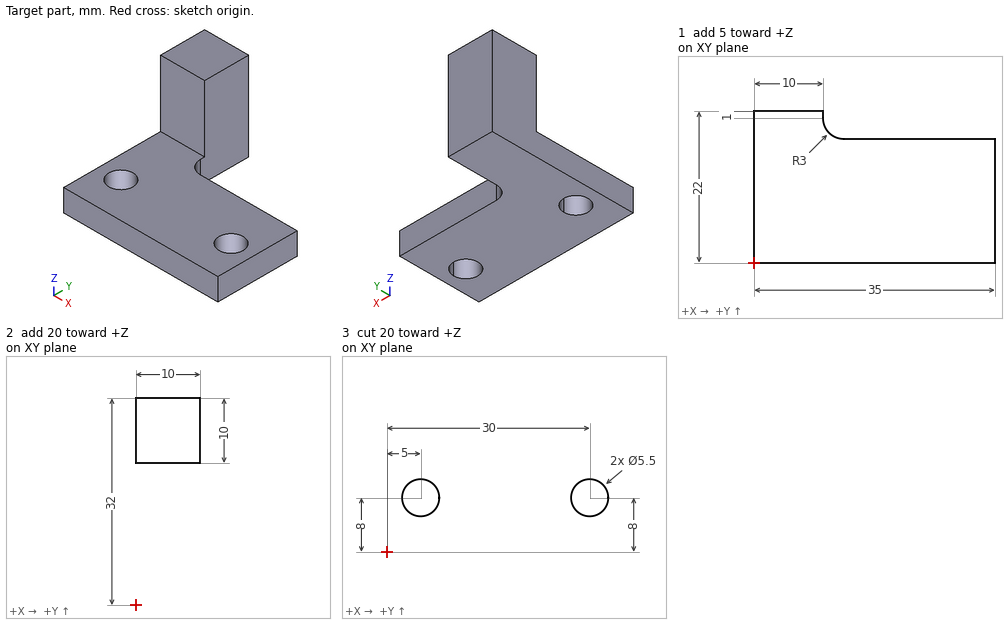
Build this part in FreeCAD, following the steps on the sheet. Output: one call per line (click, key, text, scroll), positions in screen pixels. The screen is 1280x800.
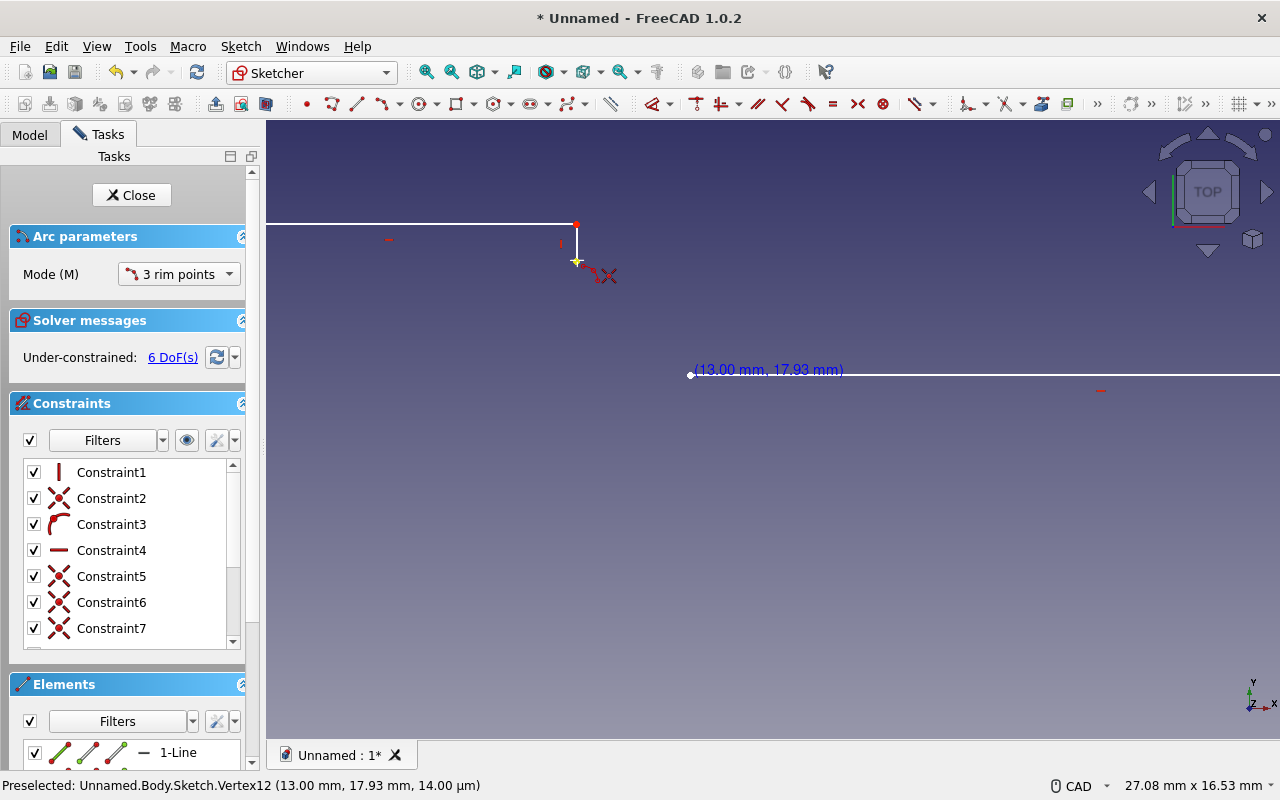
click(577, 262)
click(611, 340)
key(Escape)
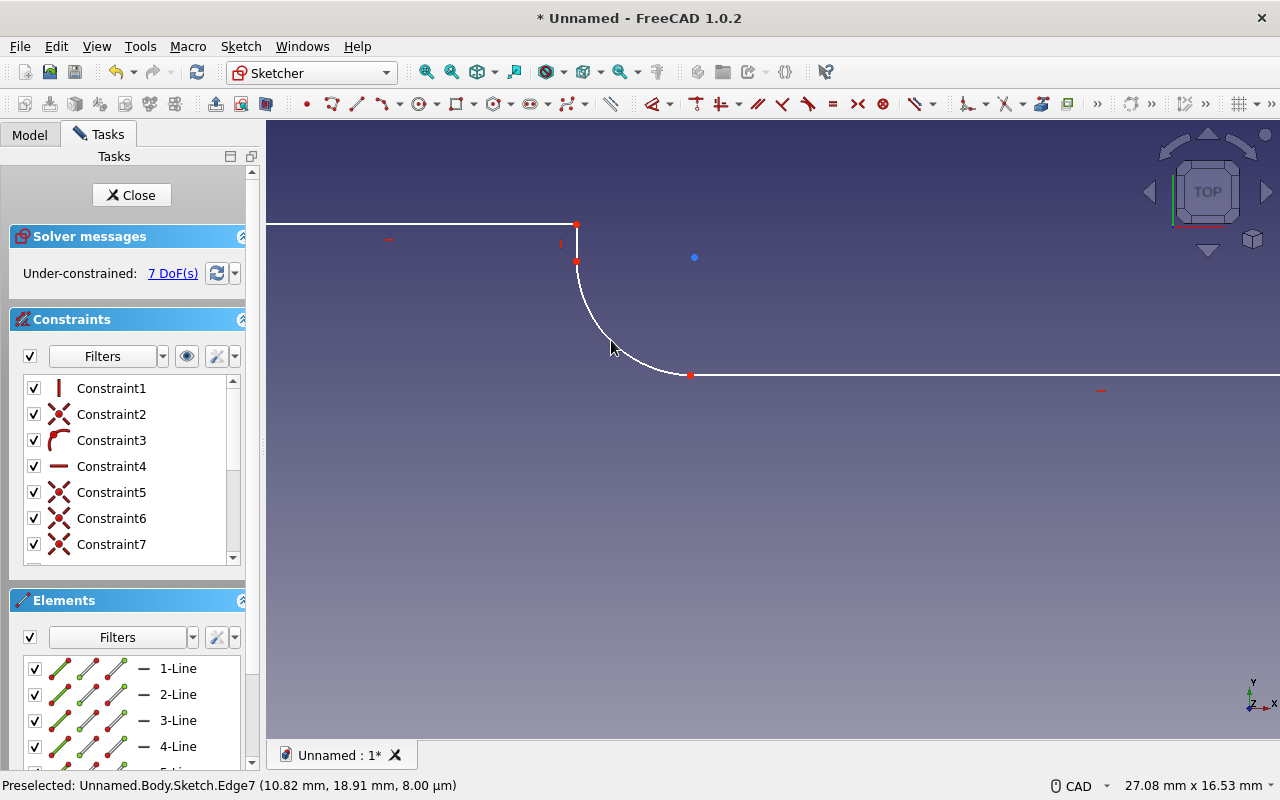
click(577, 251)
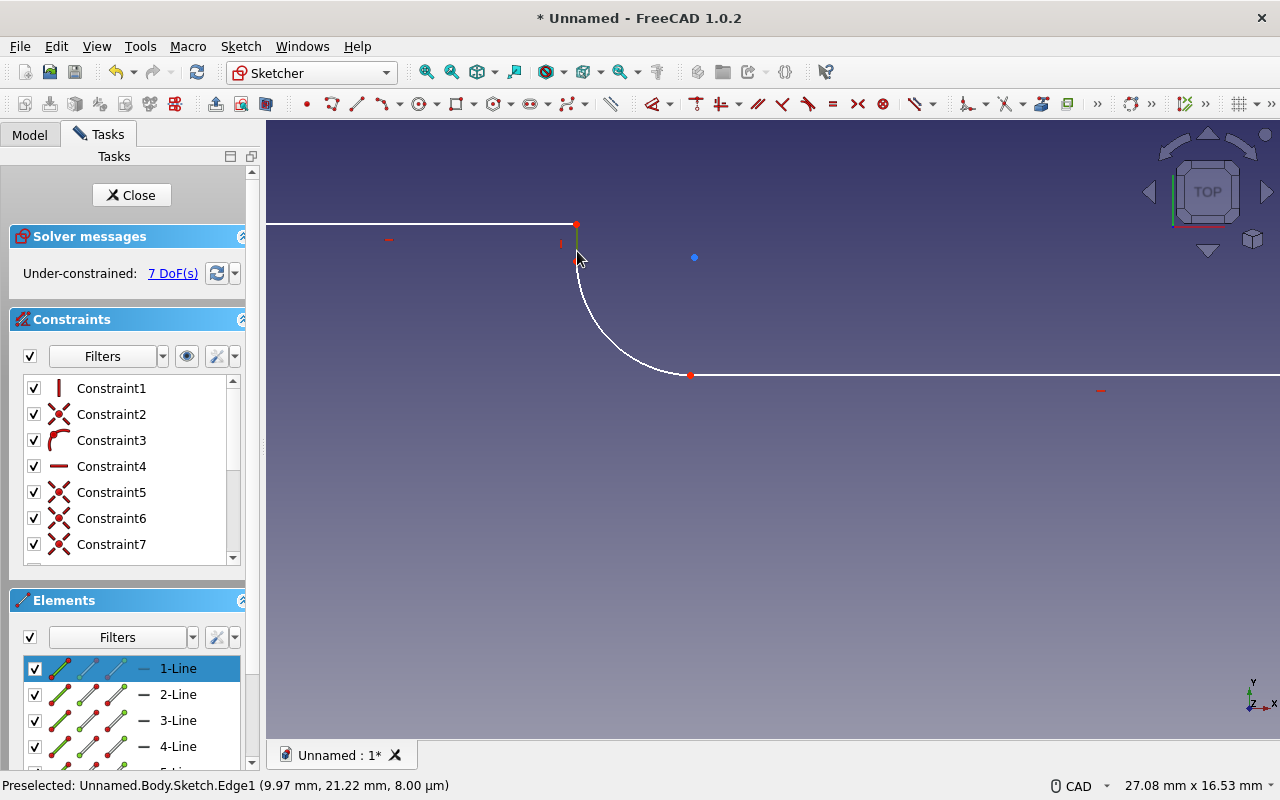
click(590, 313)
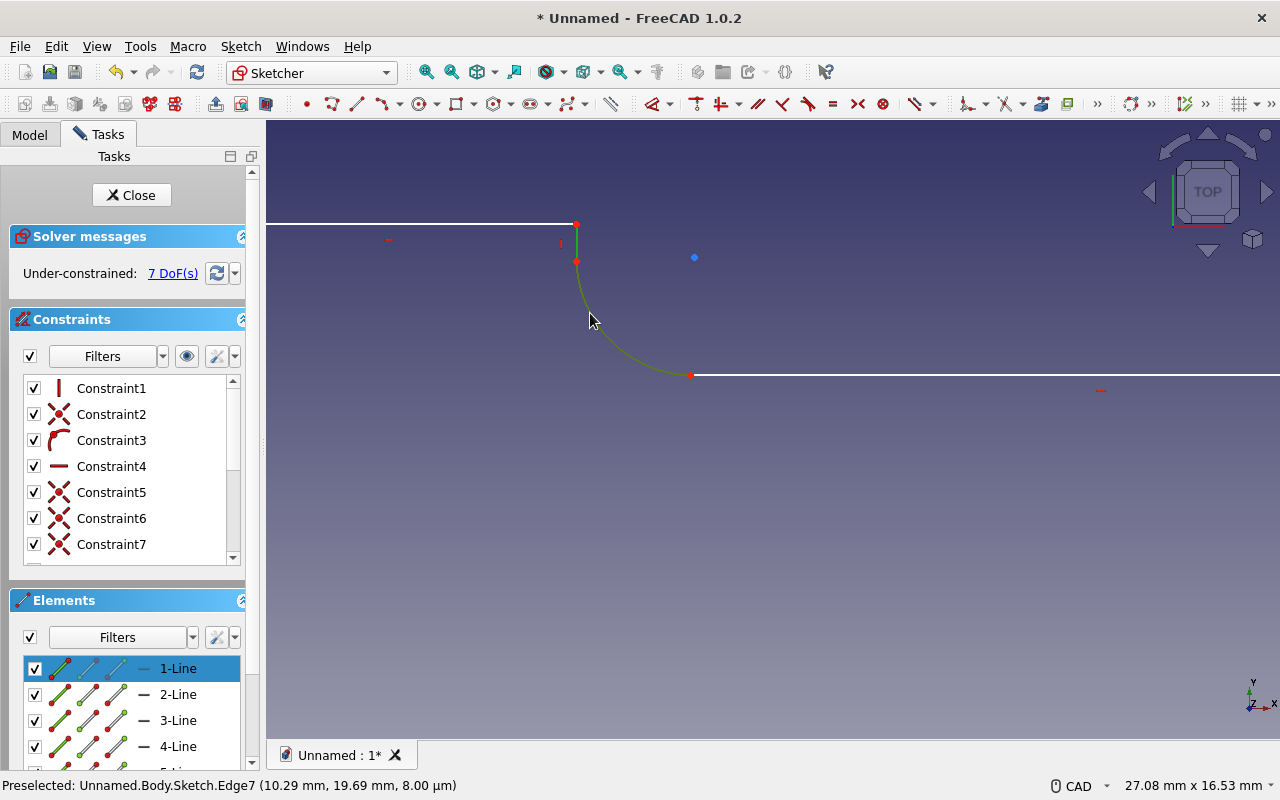
click(808, 104)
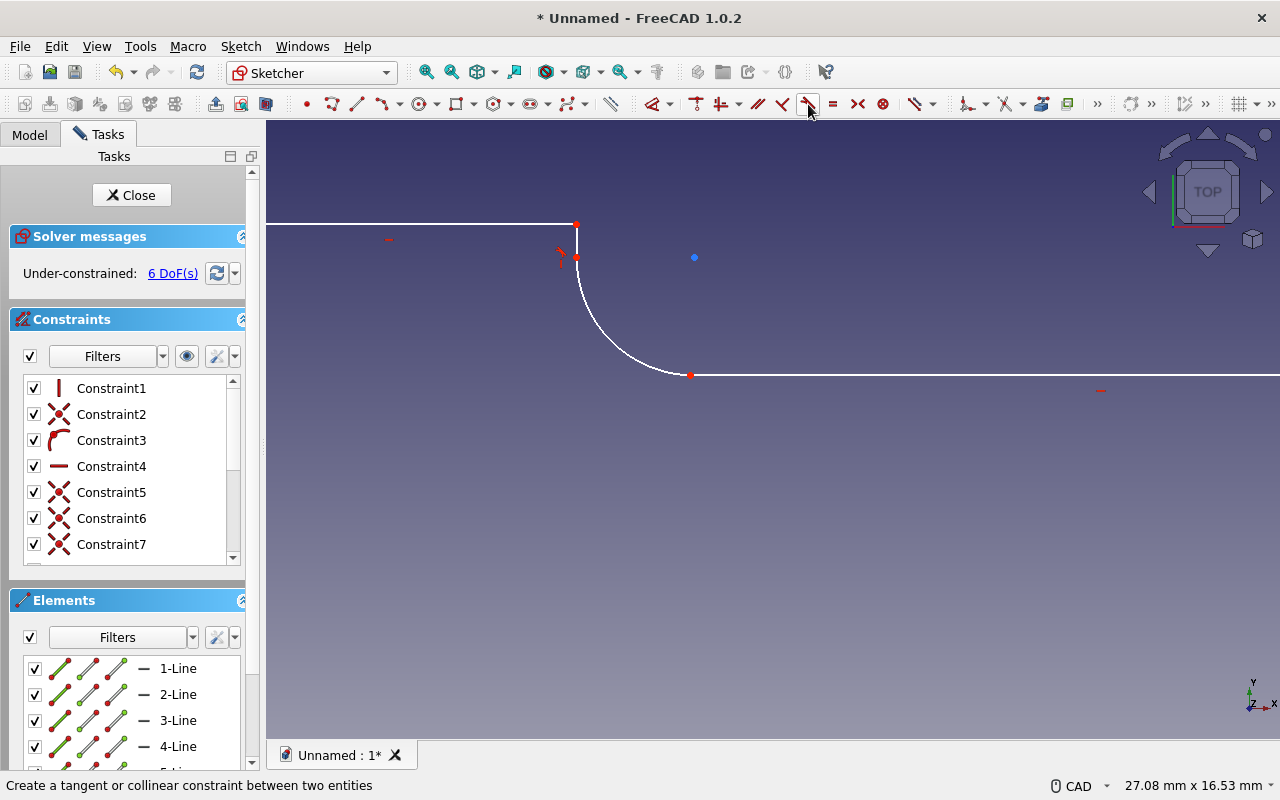
click(937, 375)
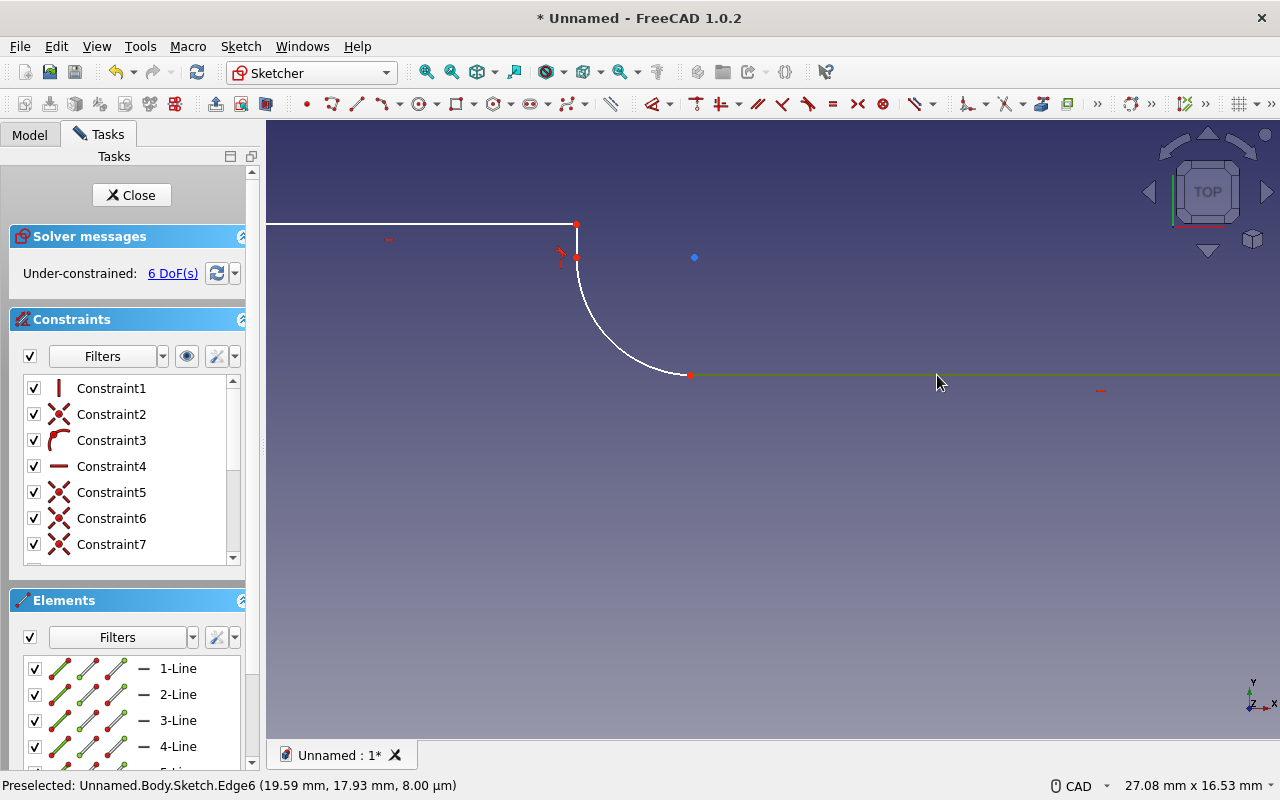
click(589, 310)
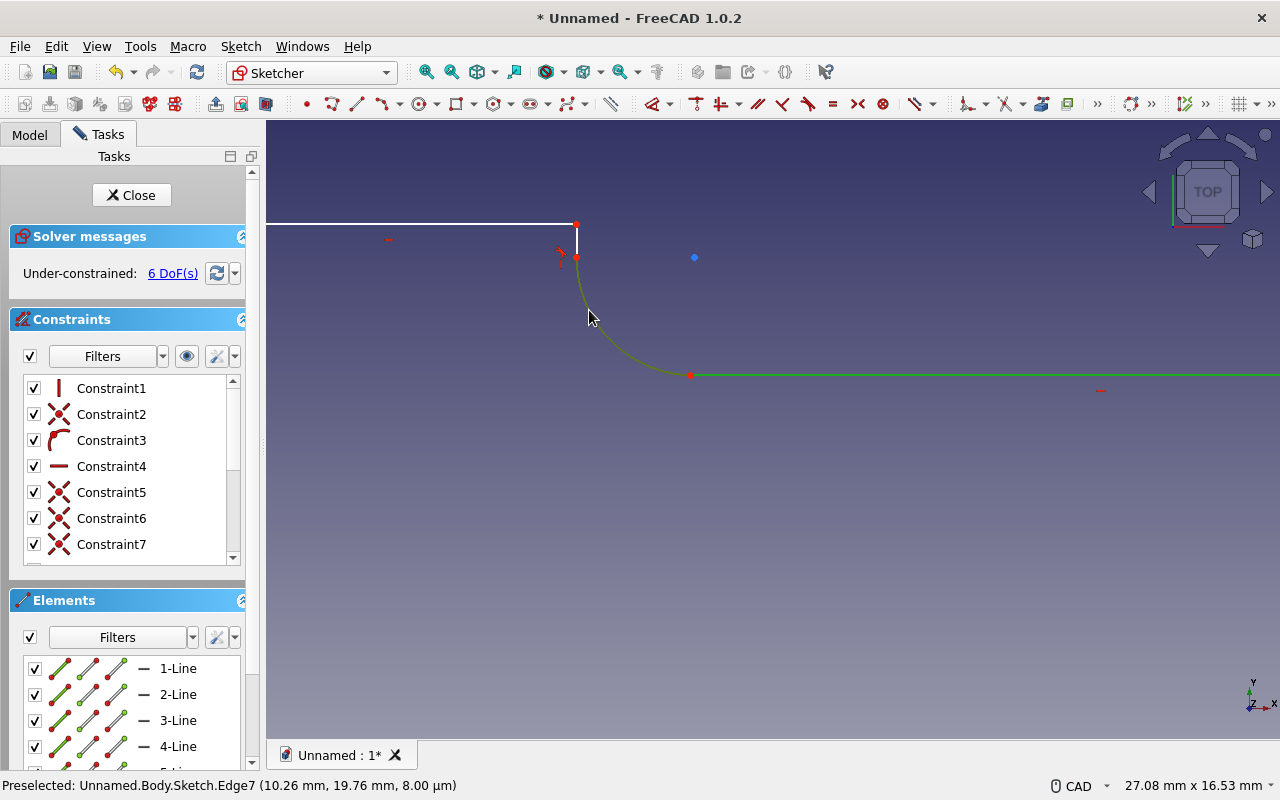
click(808, 104)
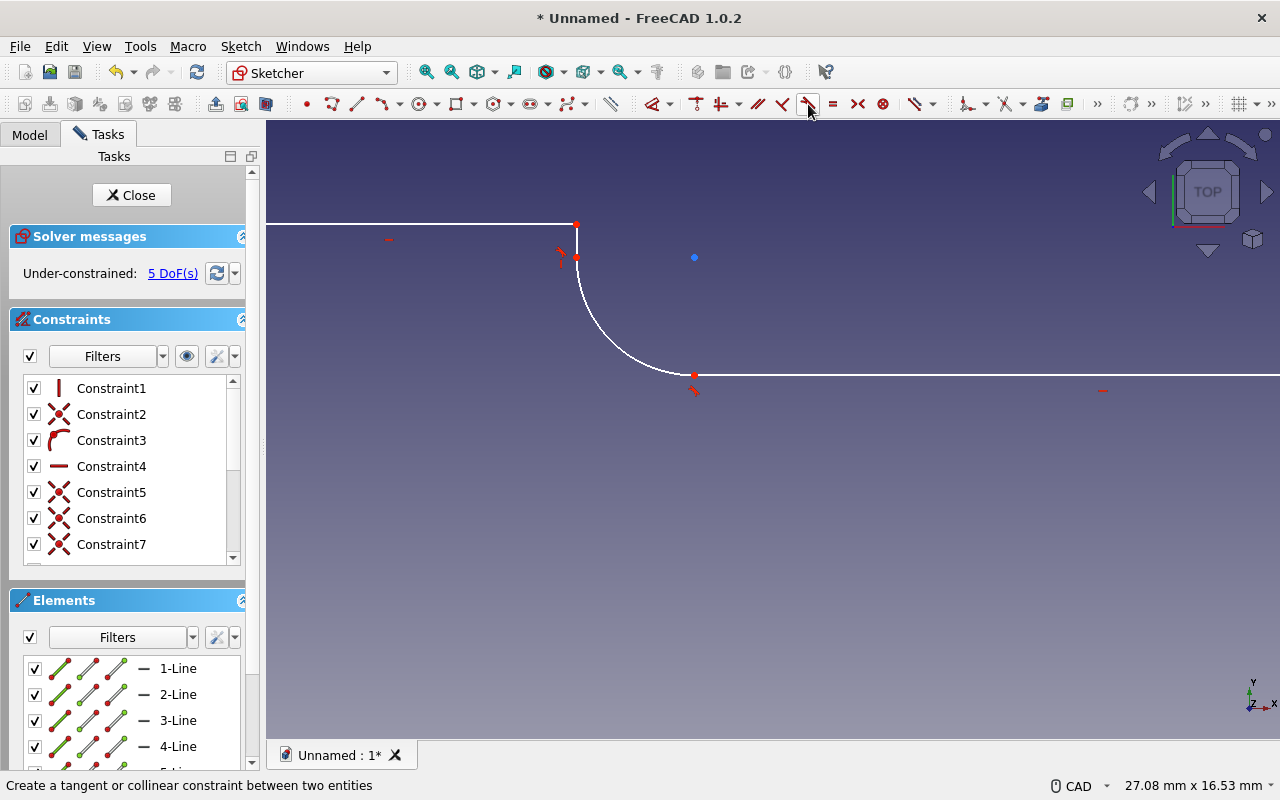
click(652, 104)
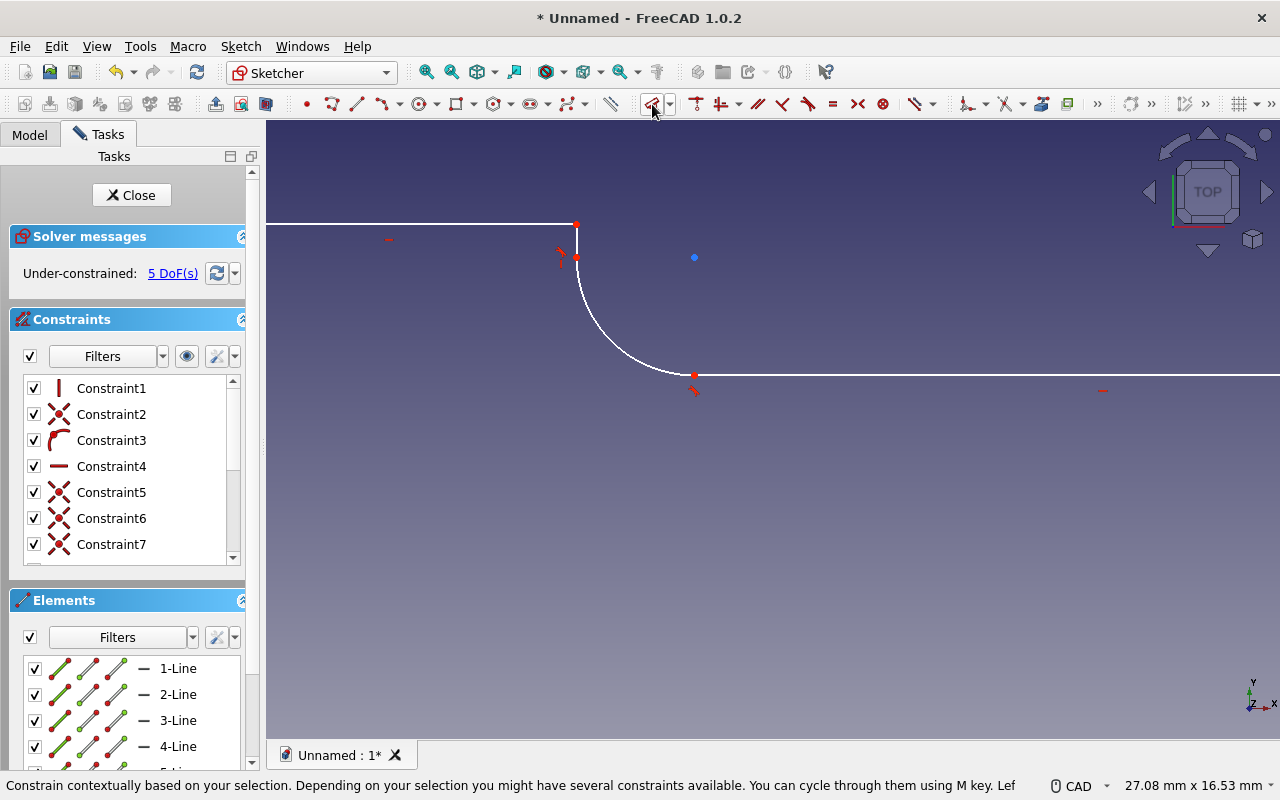
click(590, 311)
click(561, 326)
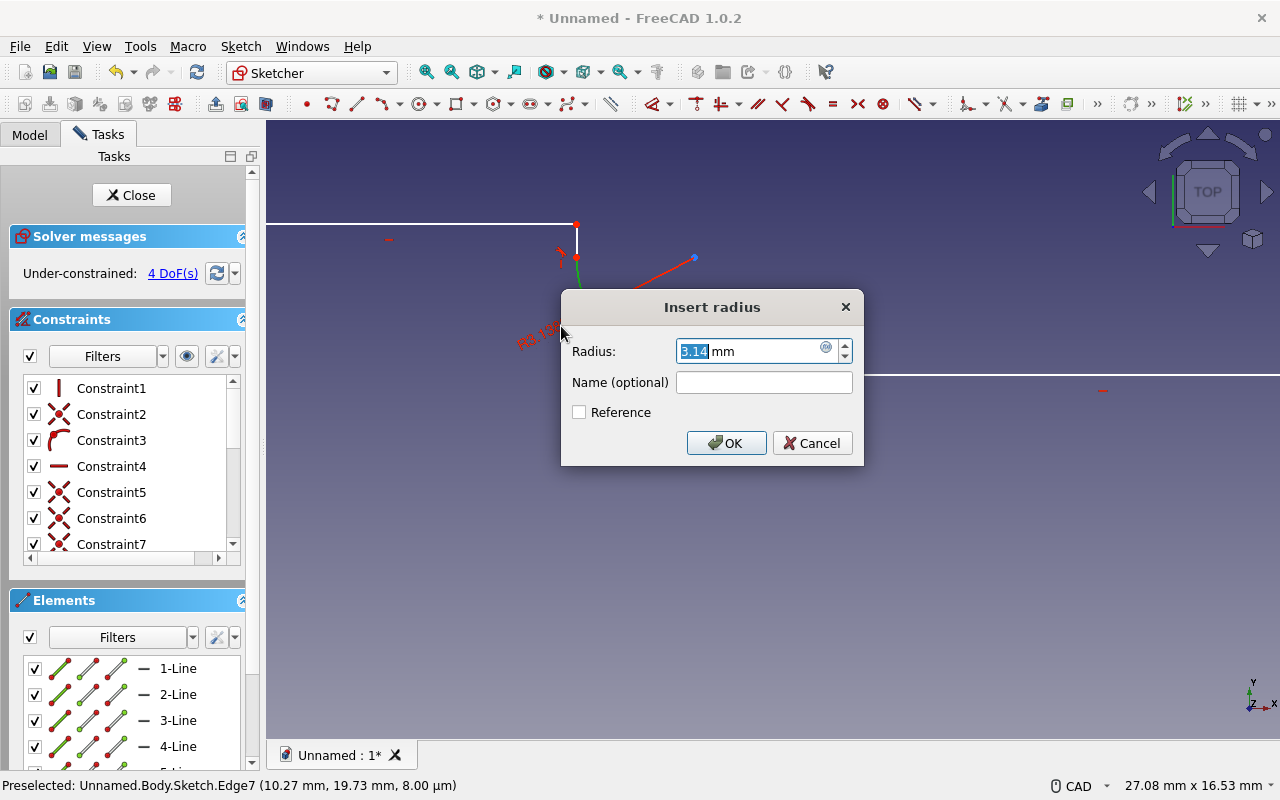
text(3)
key(Return)